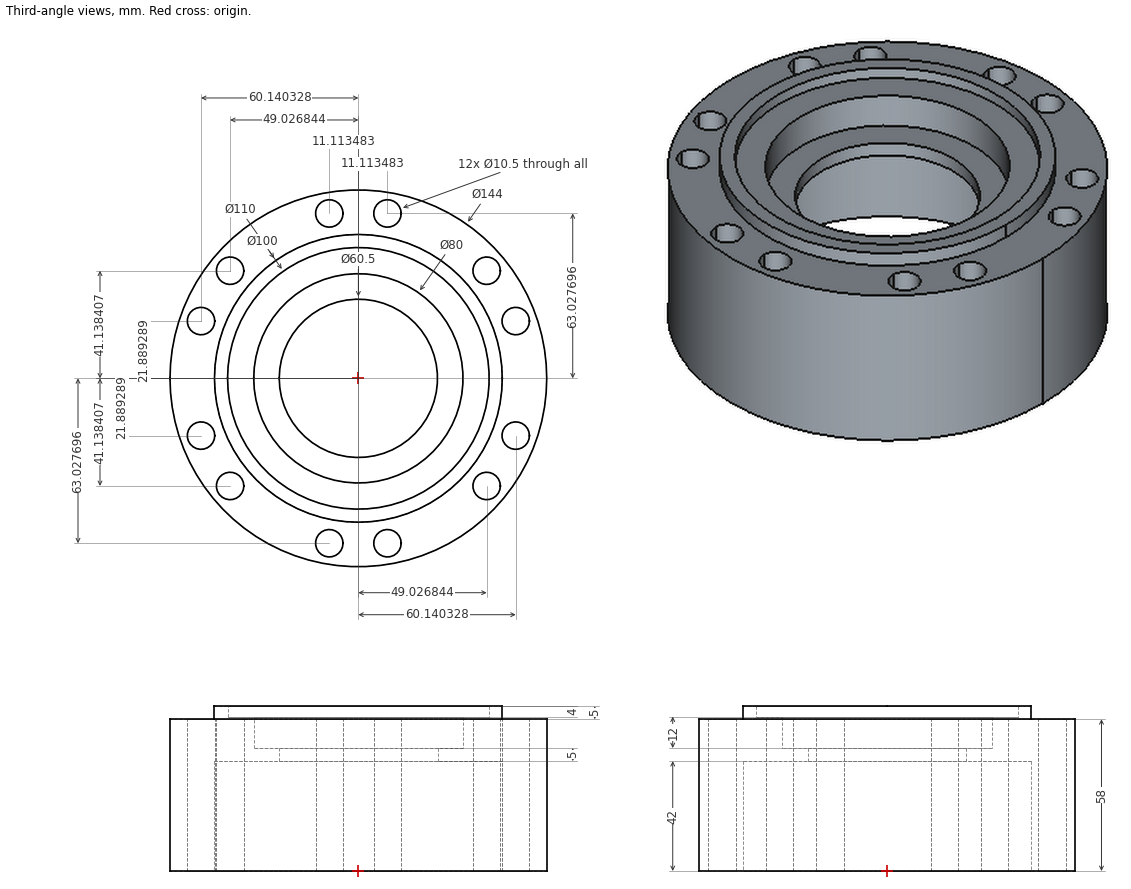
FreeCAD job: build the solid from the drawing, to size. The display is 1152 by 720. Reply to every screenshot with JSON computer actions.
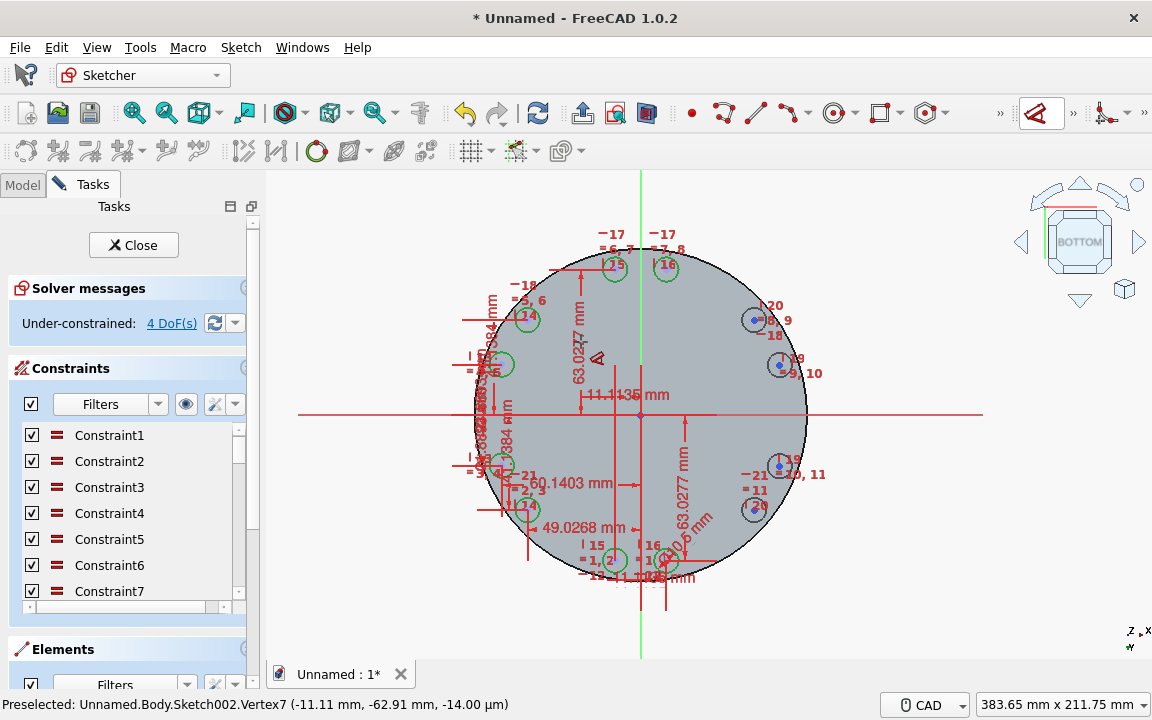
{"action": "left_click", "coordinate": [754, 320]}
{"action": "left_click", "coordinate": [697, 286]}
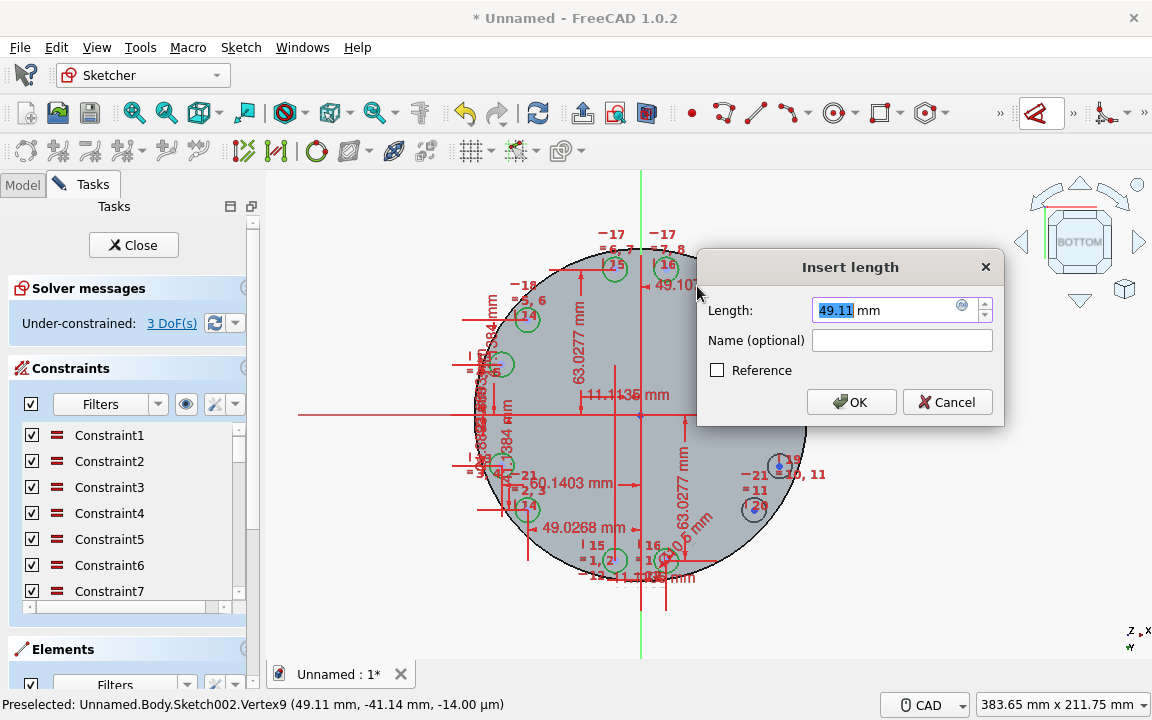
{"action": "type", "text": "49.026844"}
{"action": "key", "text": "Return"}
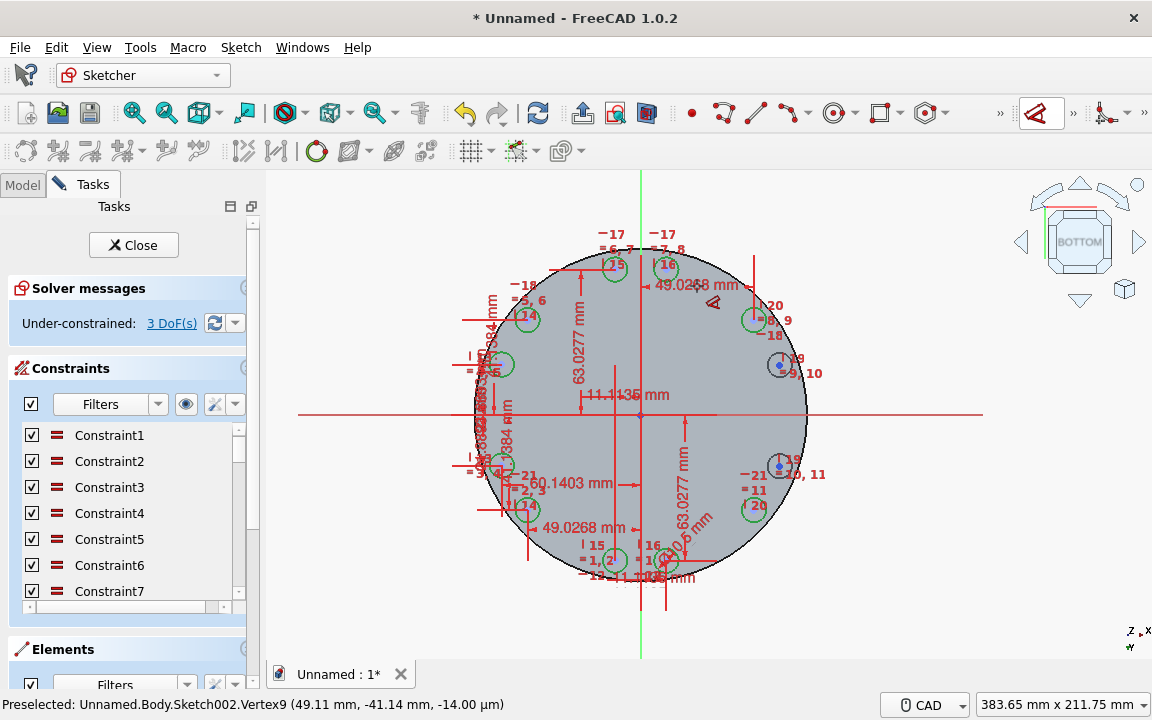
{"action": "left_click", "coordinate": [780, 365]}
{"action": "left_click", "coordinate": [710, 331]}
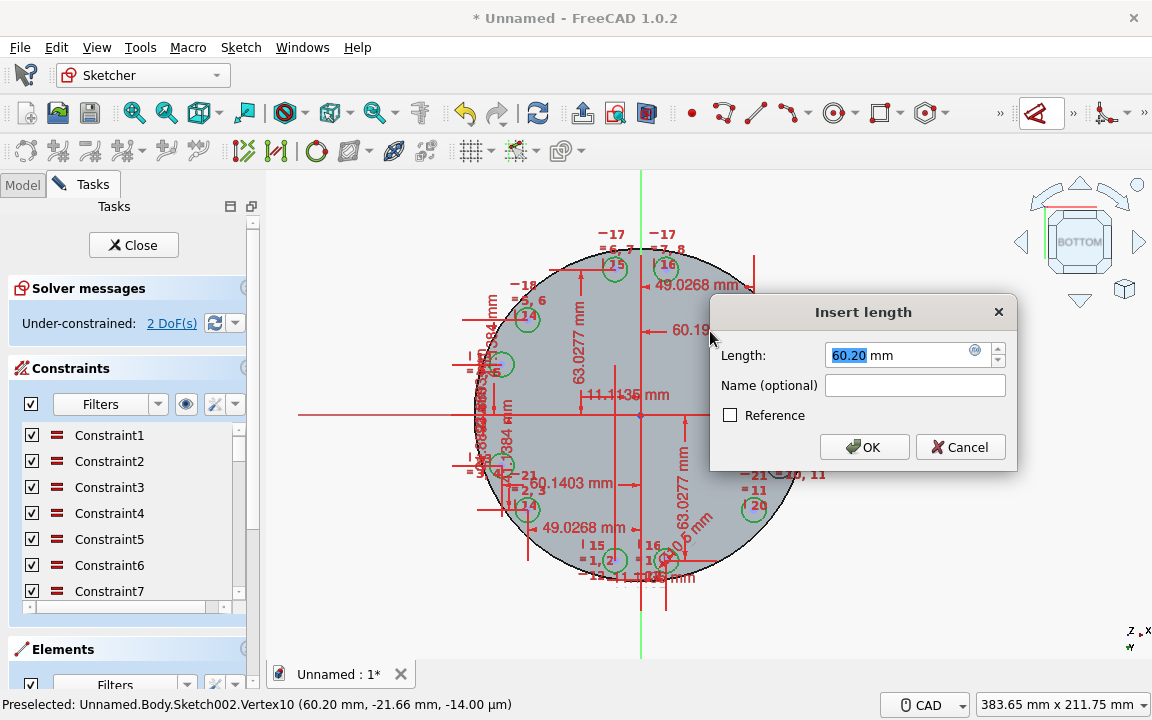
{"action": "type", "text": "60.140328"}
{"action": "key", "text": "Return"}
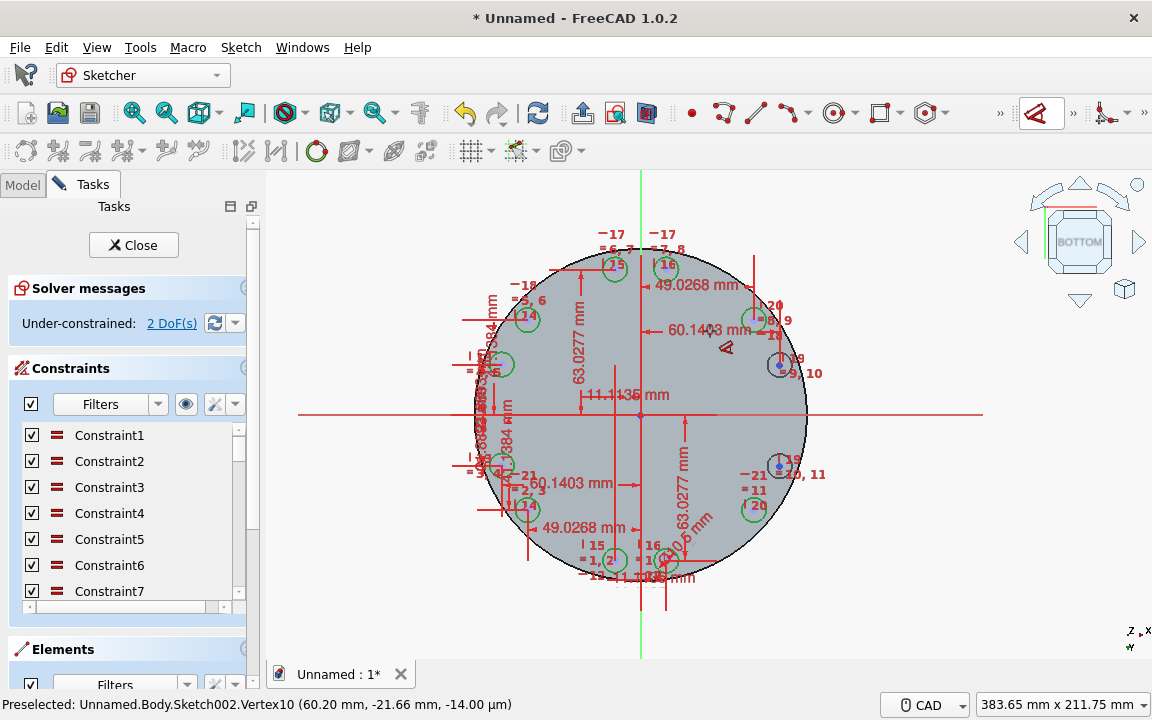
{"action": "left_click", "coordinate": [780, 365]}
{"action": "left_click", "coordinate": [814, 390]}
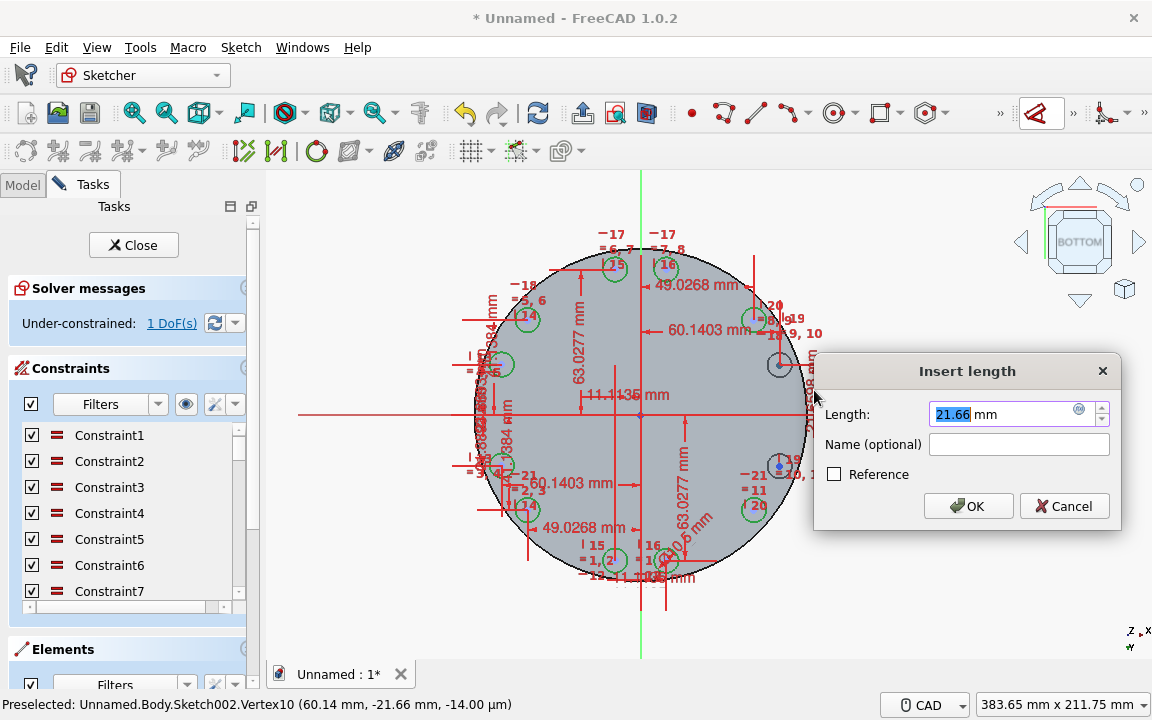
{"action": "type", "text": "21.889289"}
{"action": "key", "text": "Return"}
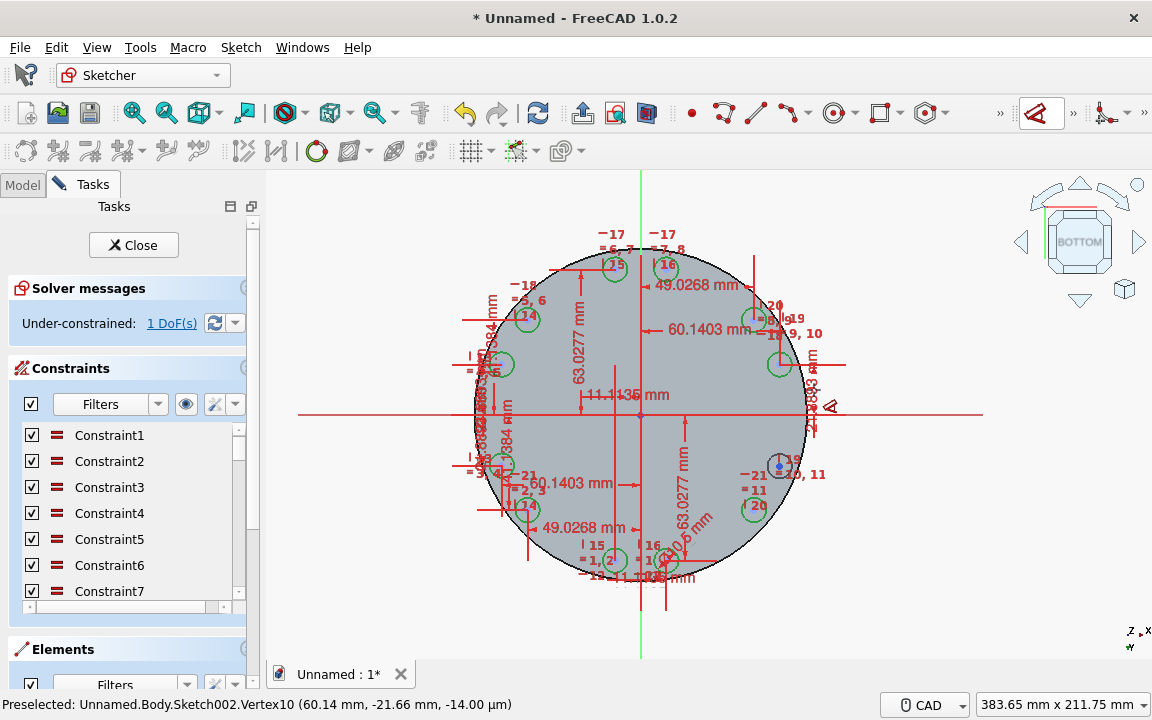
{"action": "left_click", "coordinate": [780, 466]}
{"action": "left_click", "coordinate": [814, 441]}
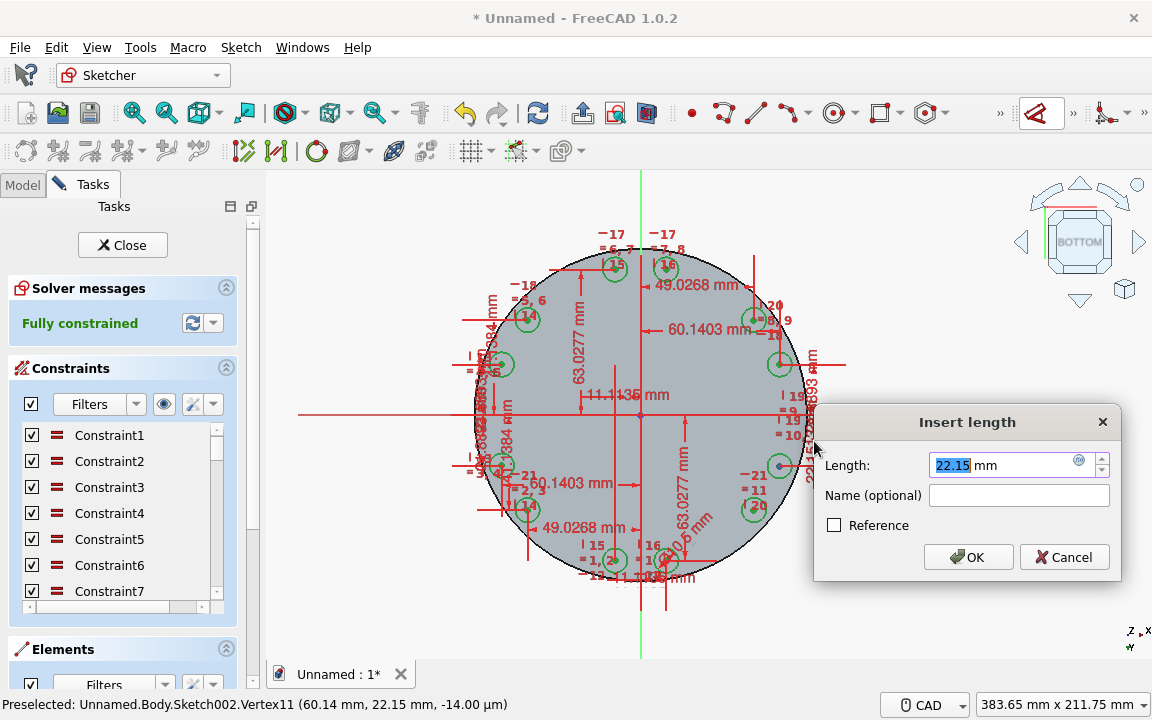
{"action": "type", "text": "21.889289"}
{"action": "key", "text": "Return"}
{"action": "key", "text": "Escape"}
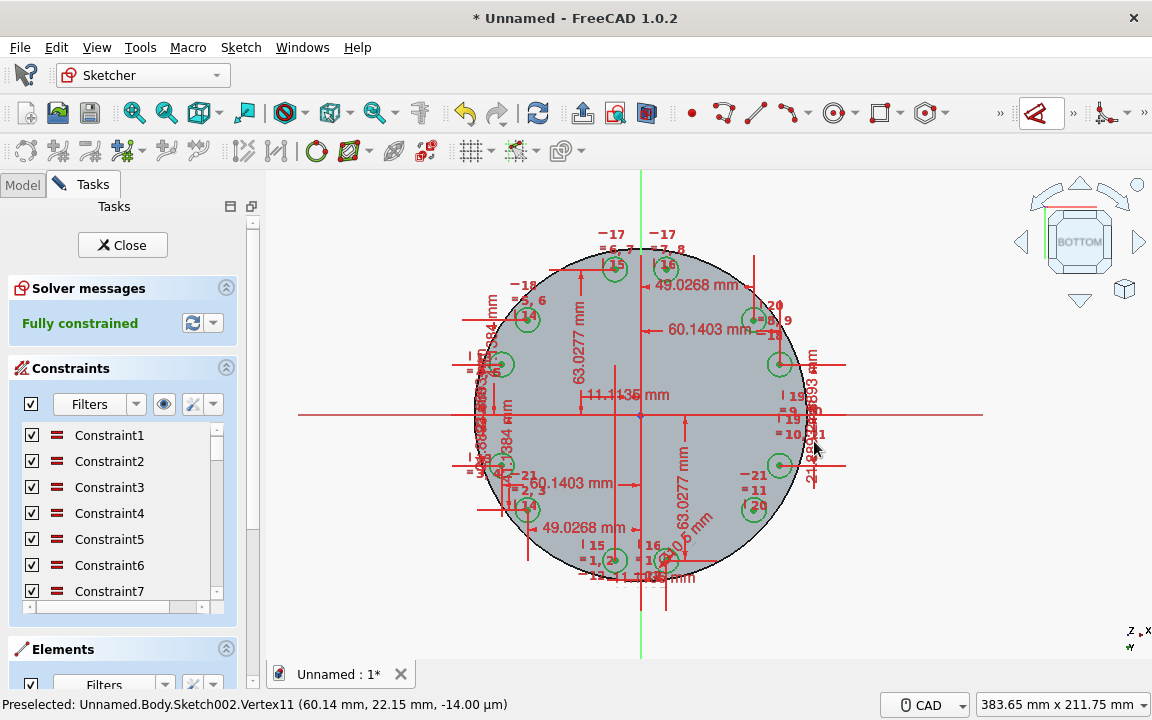
{"action": "left_click", "coordinate": [123, 245]}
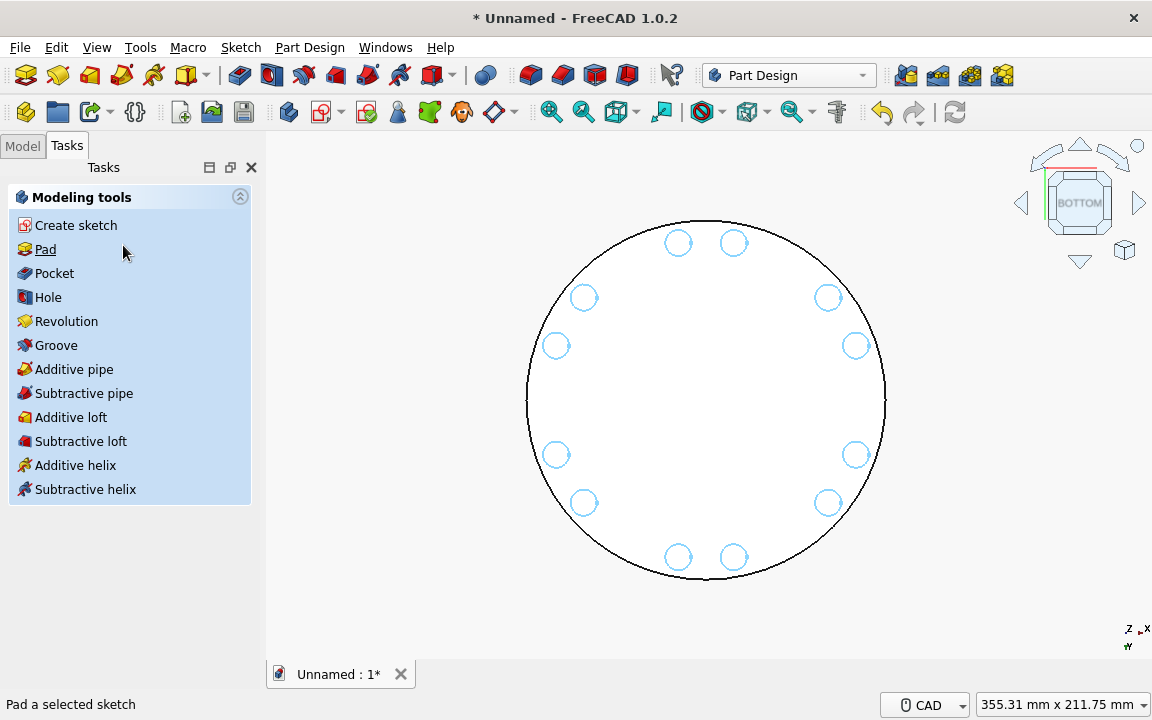
{"action": "left_click", "coordinate": [272, 76]}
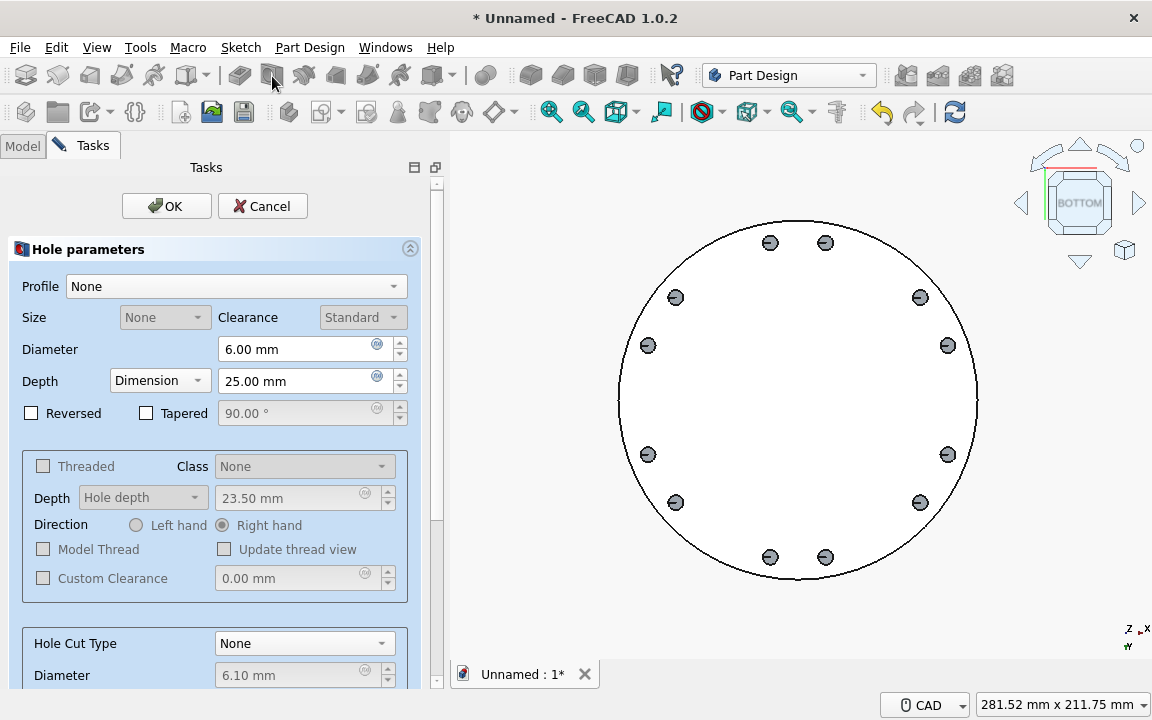
{"action": "triple_click", "coordinate": [305, 349]}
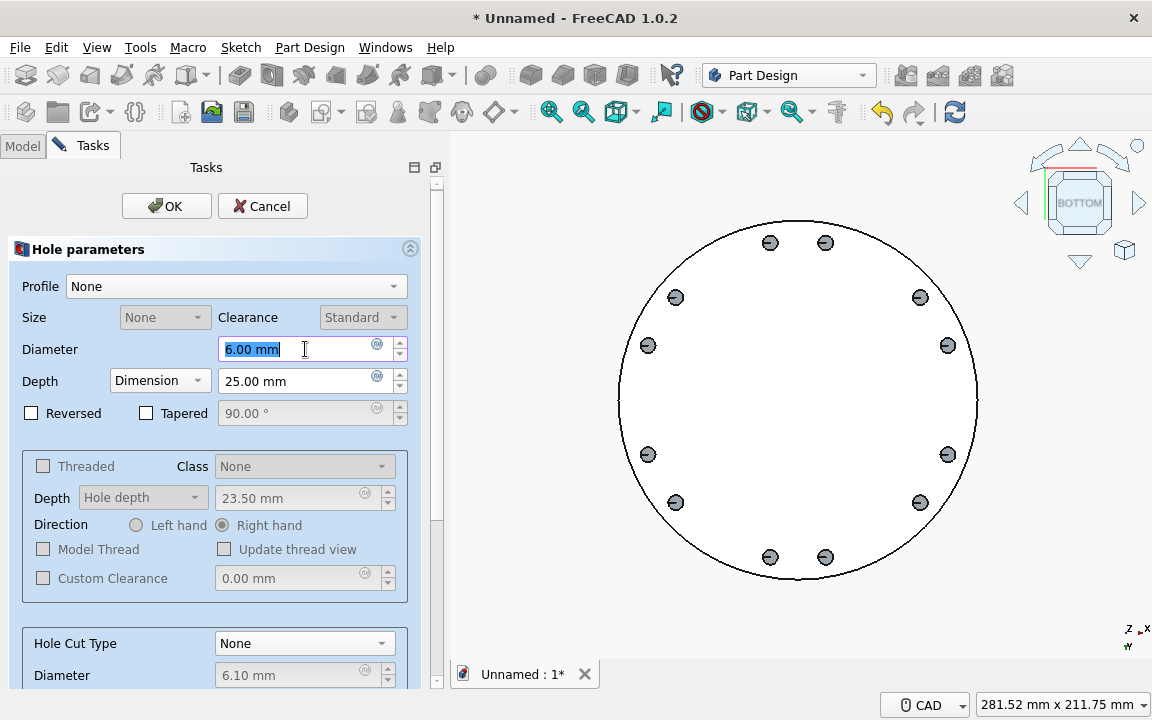
{"action": "type", "text": "10.5"}
{"action": "key", "text": "Tab"}